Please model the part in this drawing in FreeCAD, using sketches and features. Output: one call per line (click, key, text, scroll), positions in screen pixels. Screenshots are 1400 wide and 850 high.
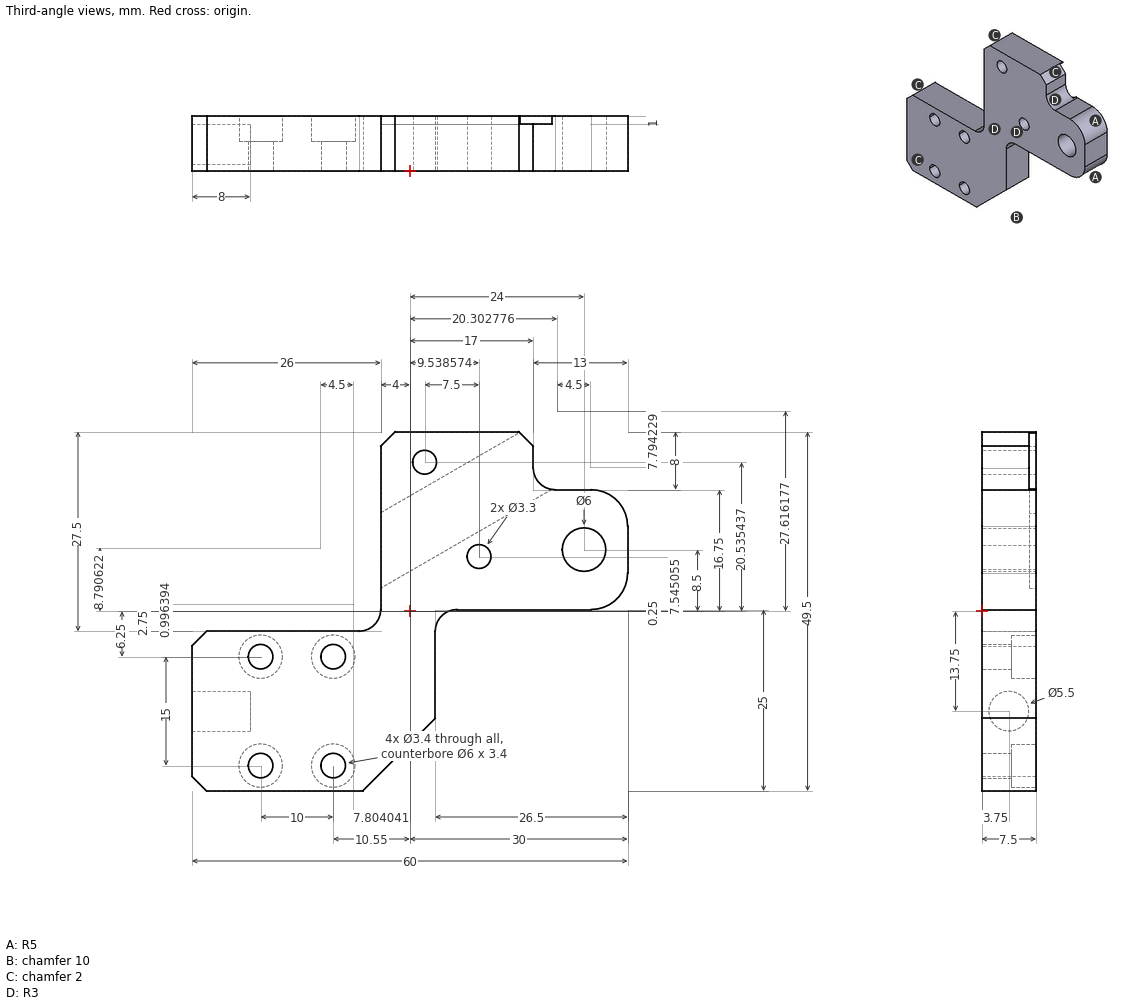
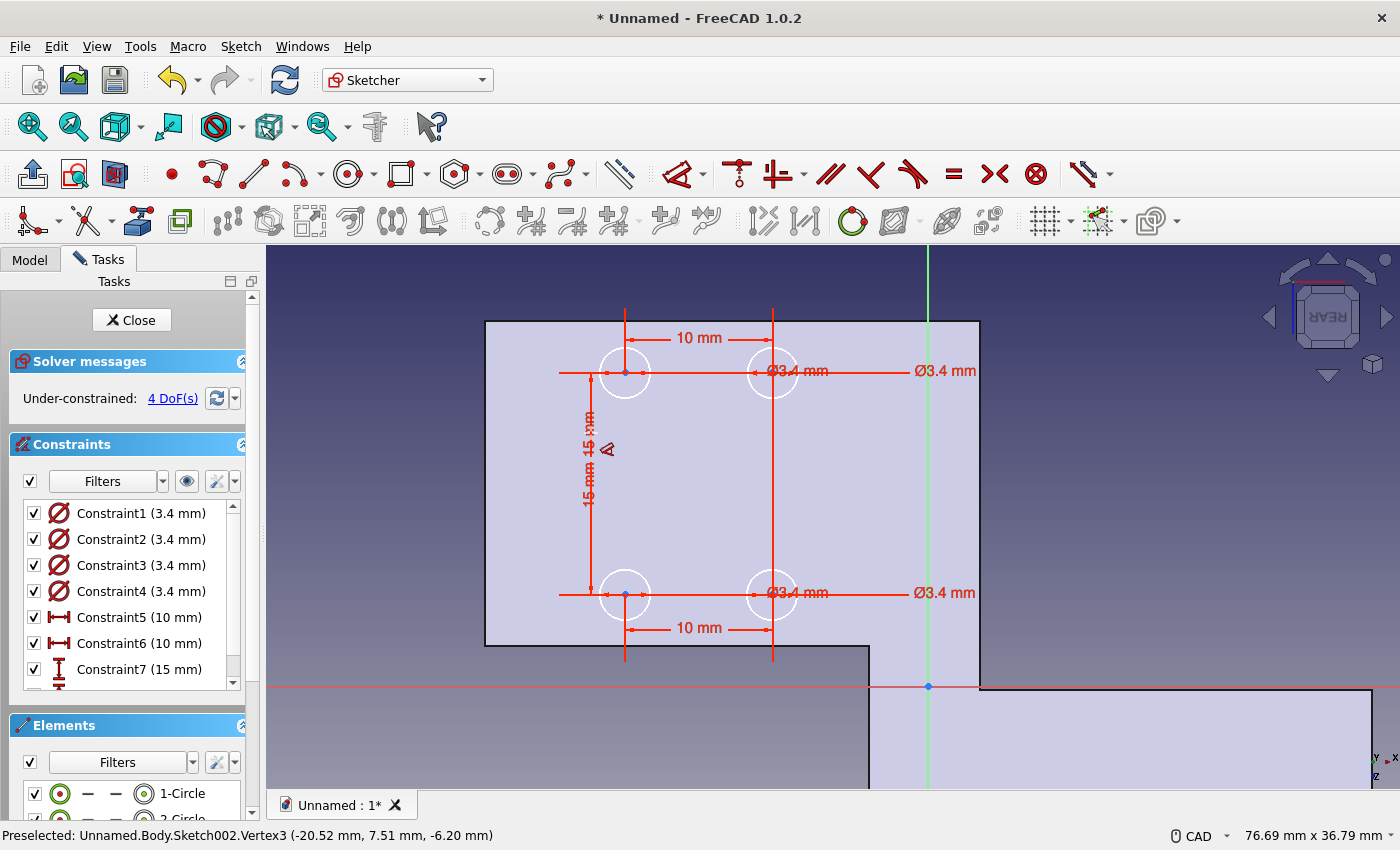
click(625, 595)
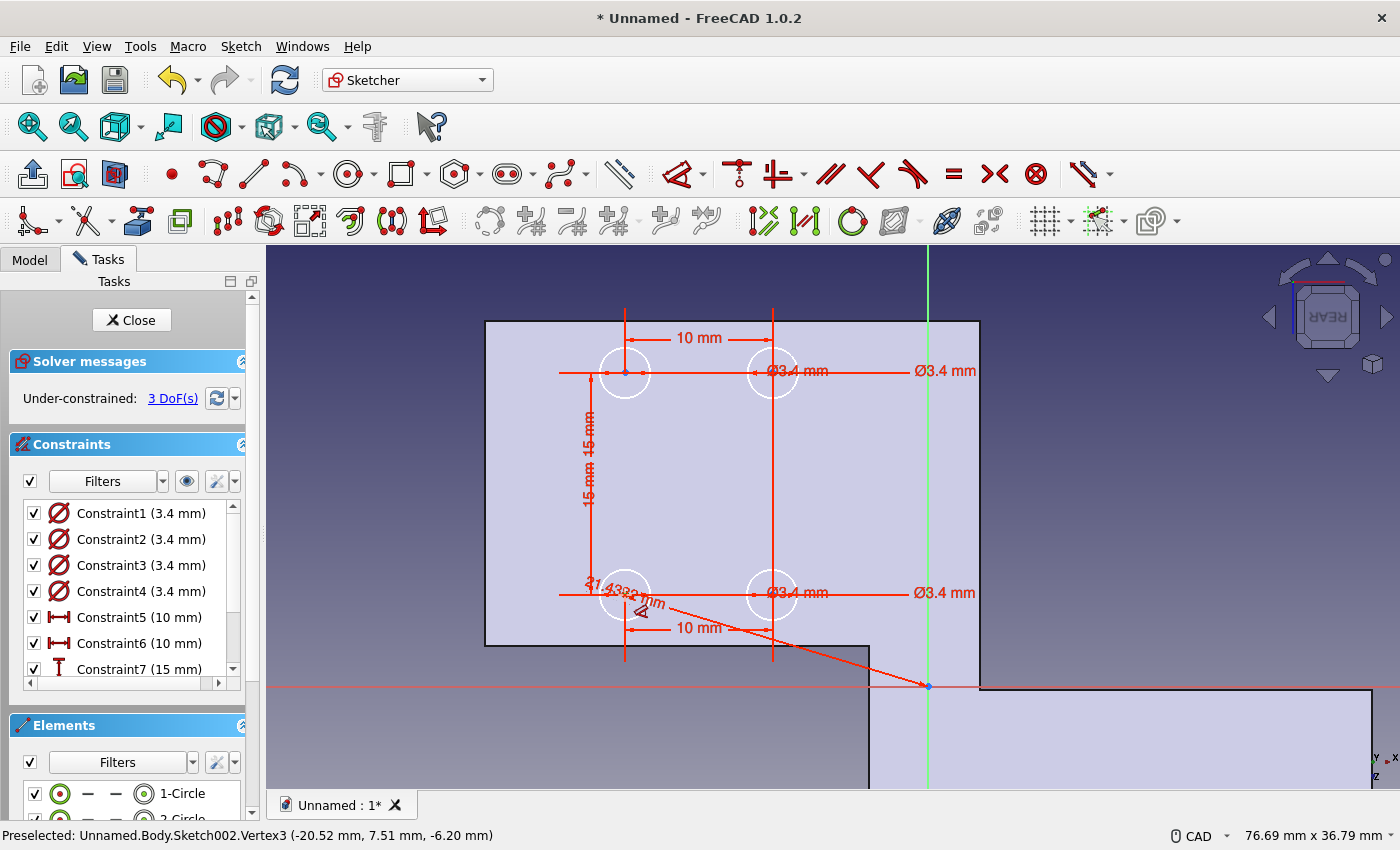
click(772, 595)
click(699, 561)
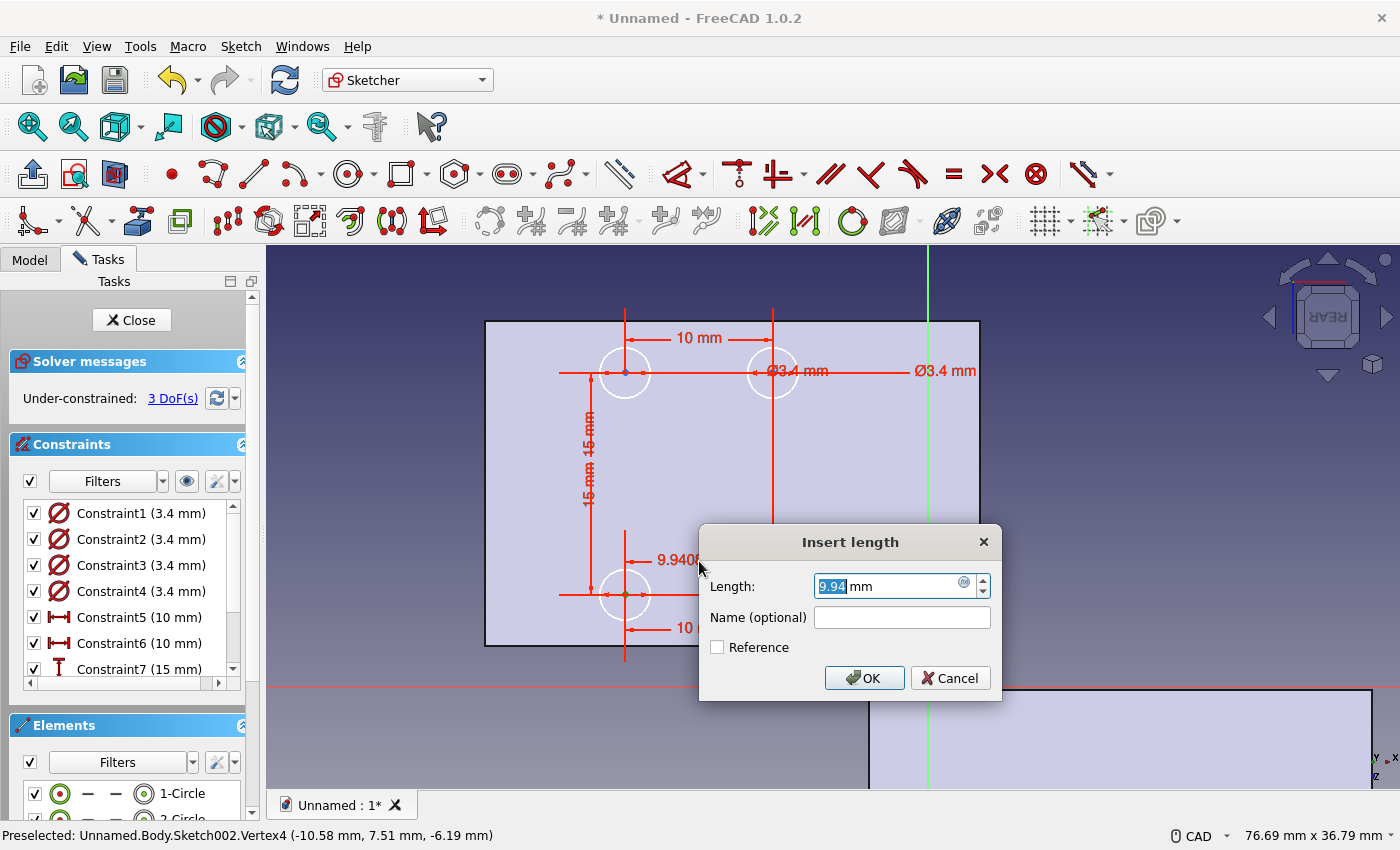
text(10)
key(Return)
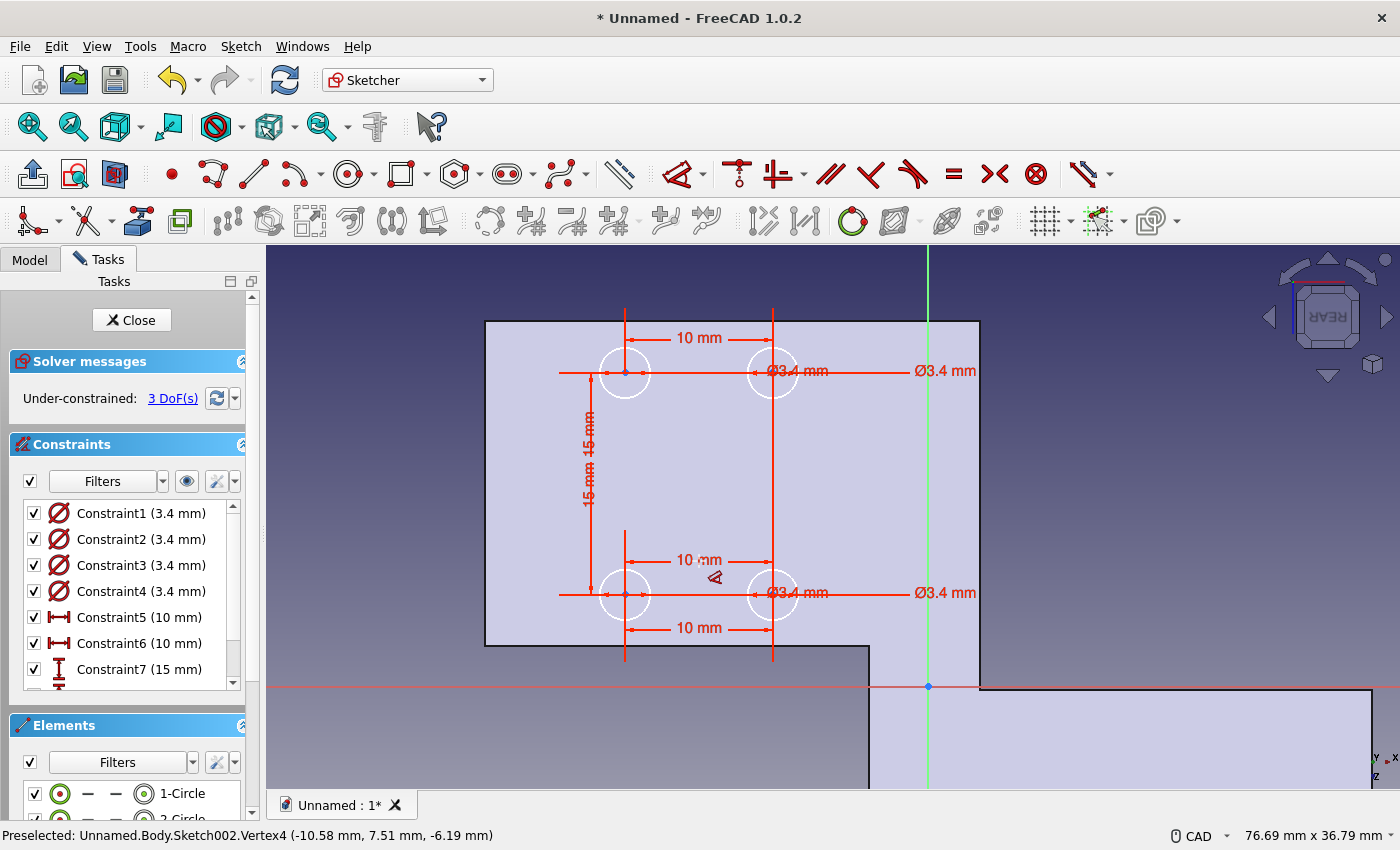
click(773, 373)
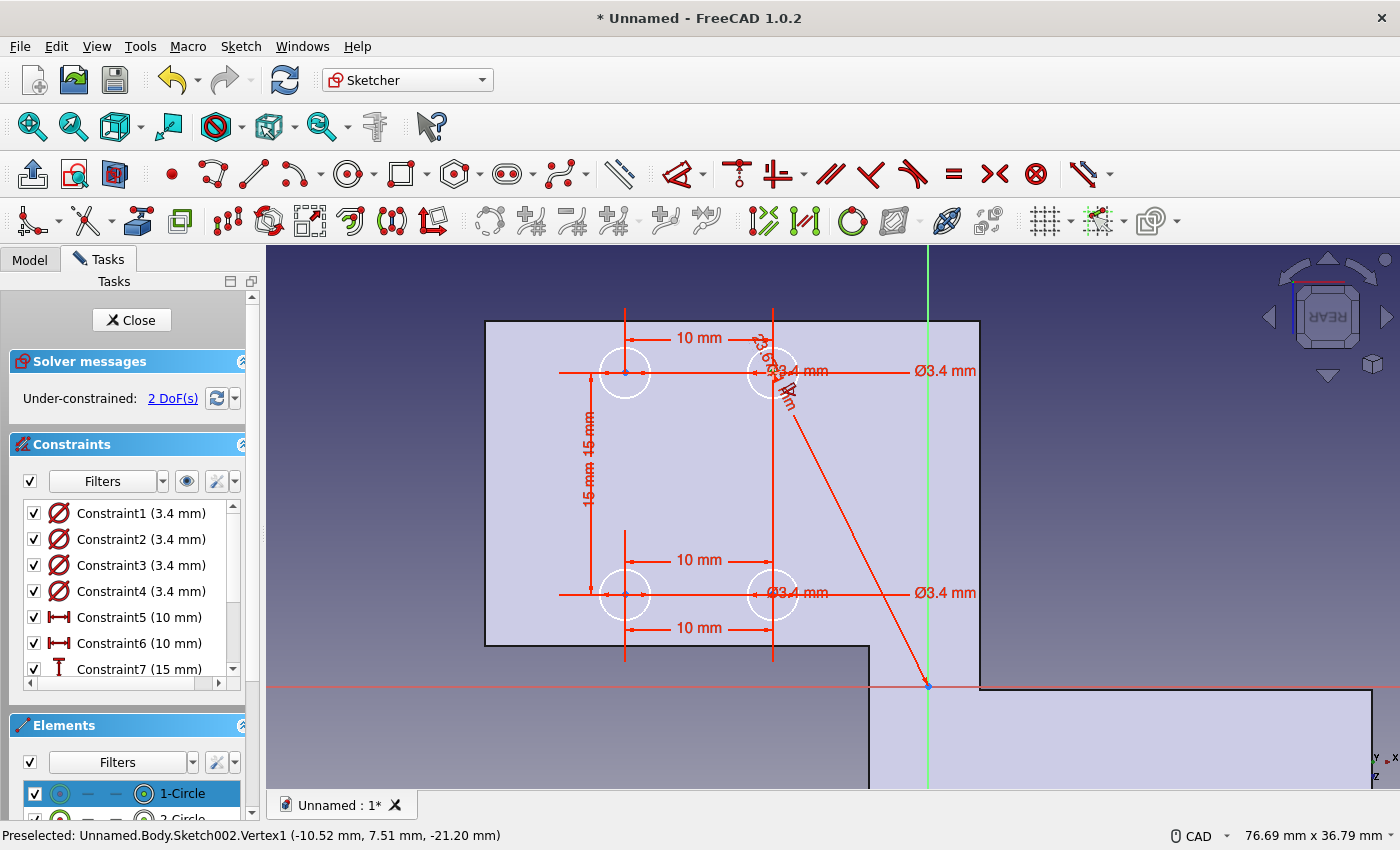
click(773, 595)
click(807, 484)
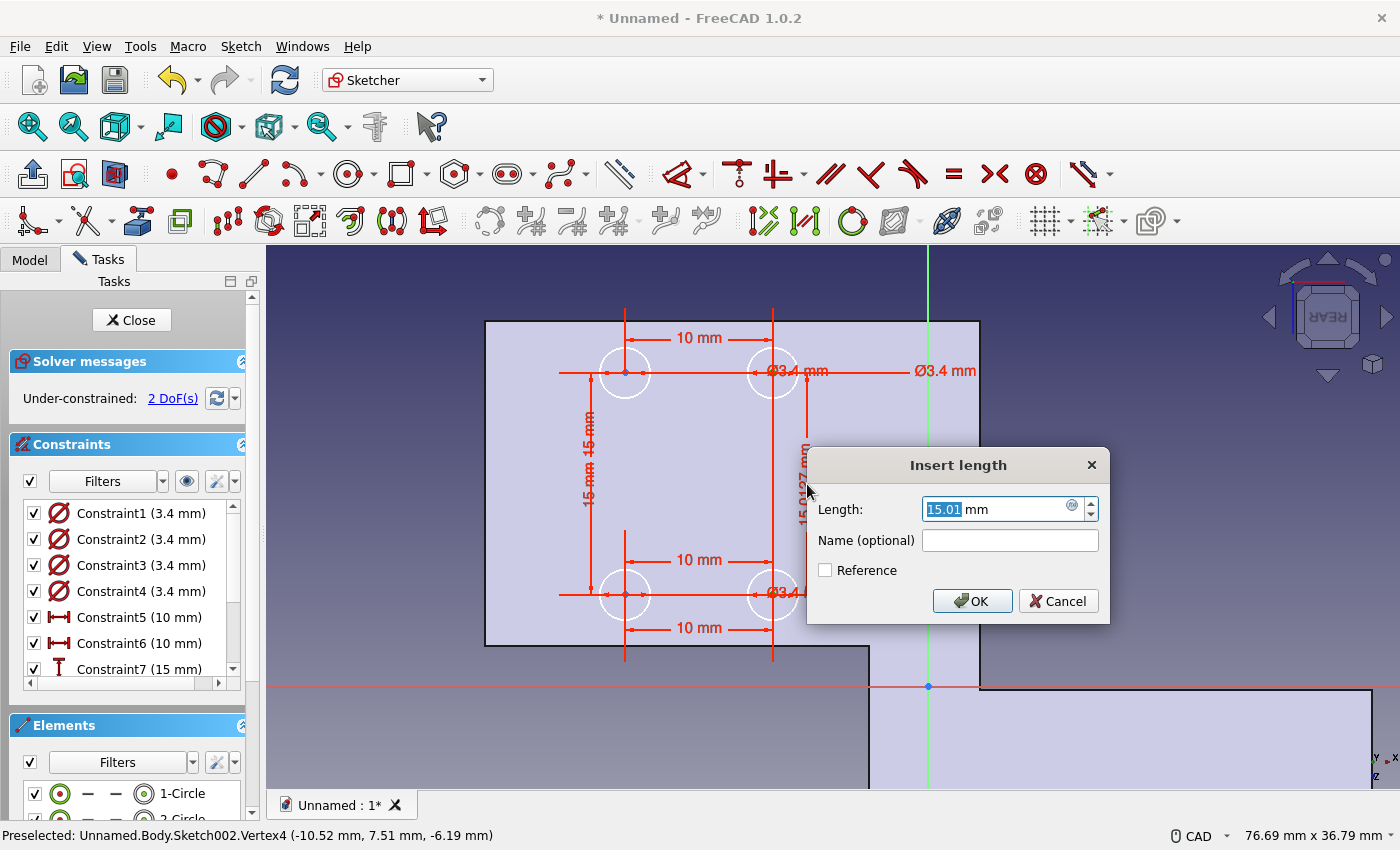
text(15)
key(Return)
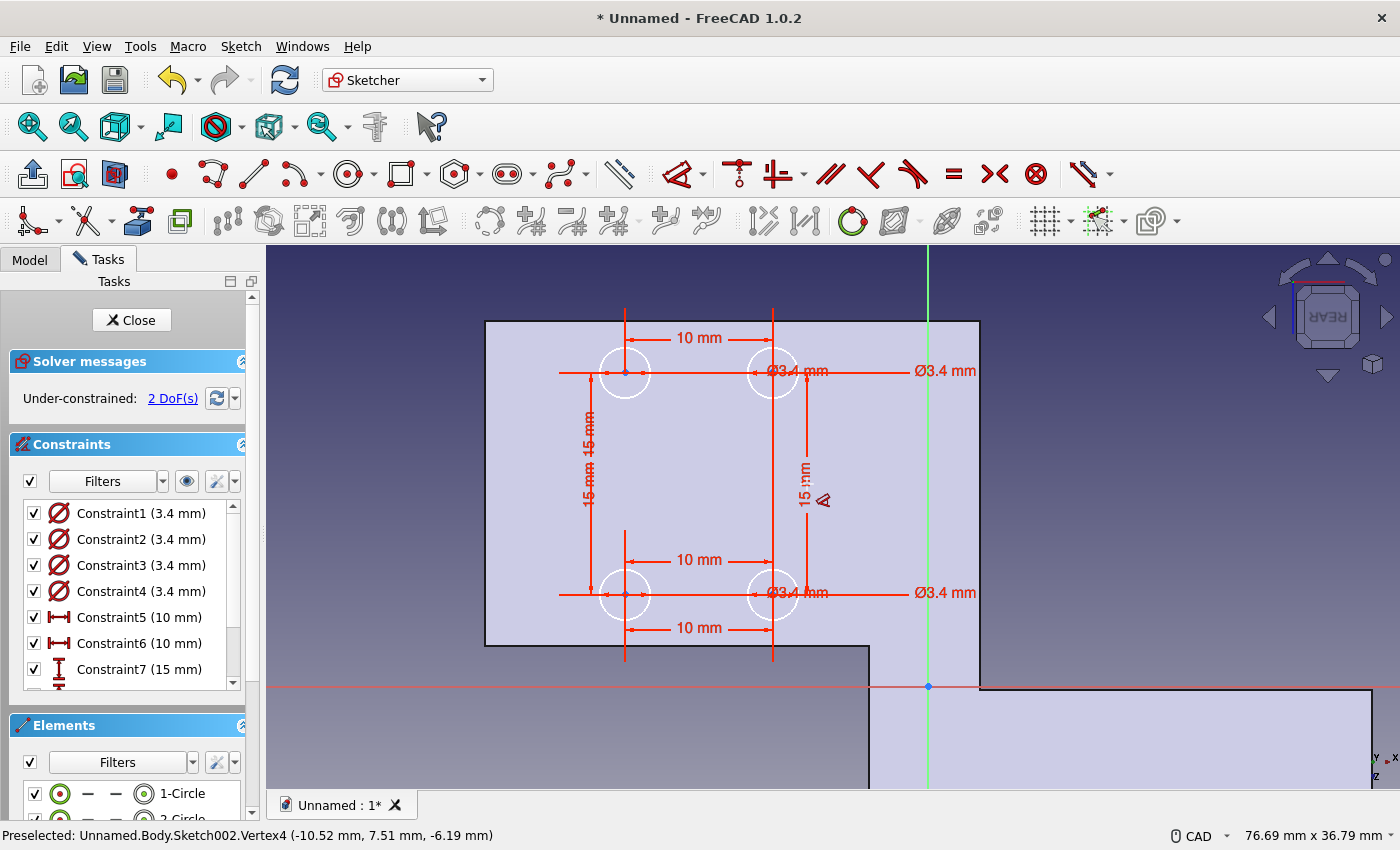
click(625, 595)
click(962, 641)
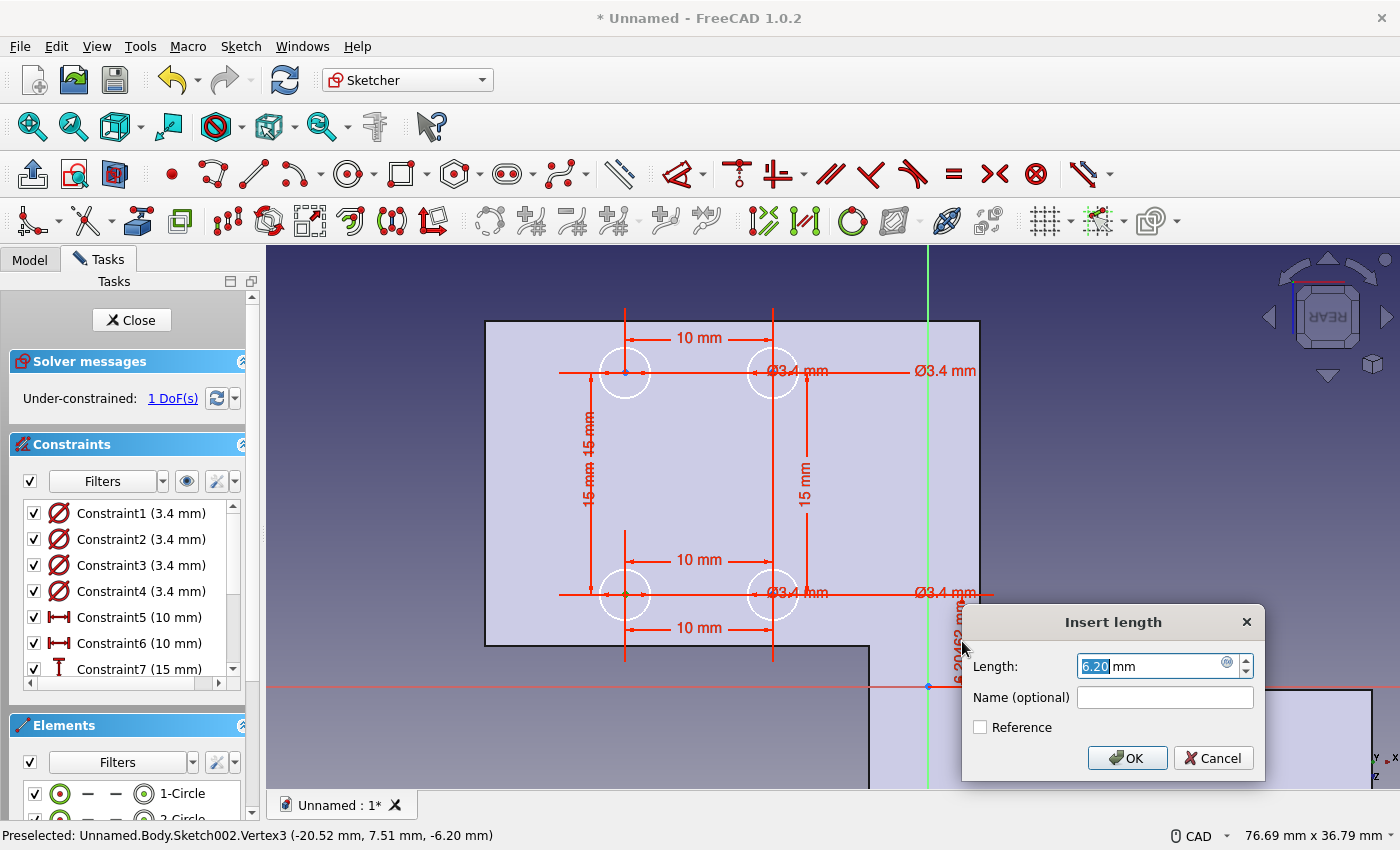
text(6.25)
key(Return)